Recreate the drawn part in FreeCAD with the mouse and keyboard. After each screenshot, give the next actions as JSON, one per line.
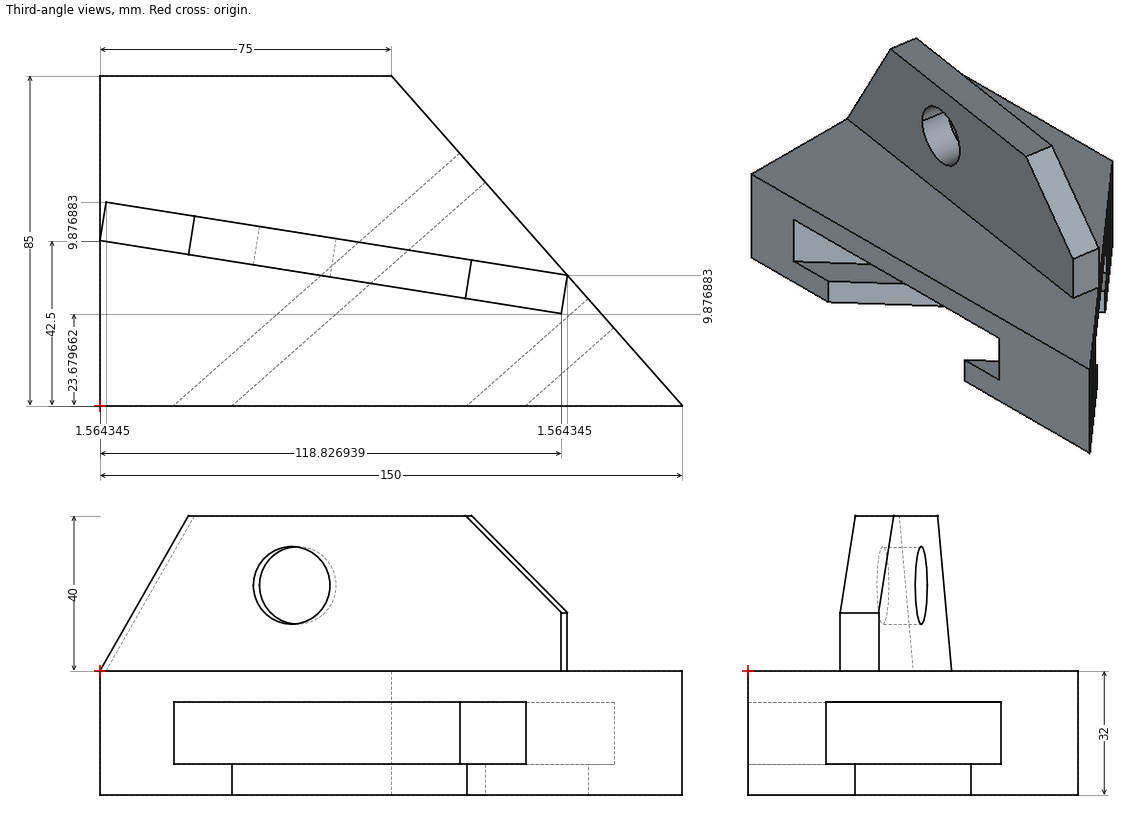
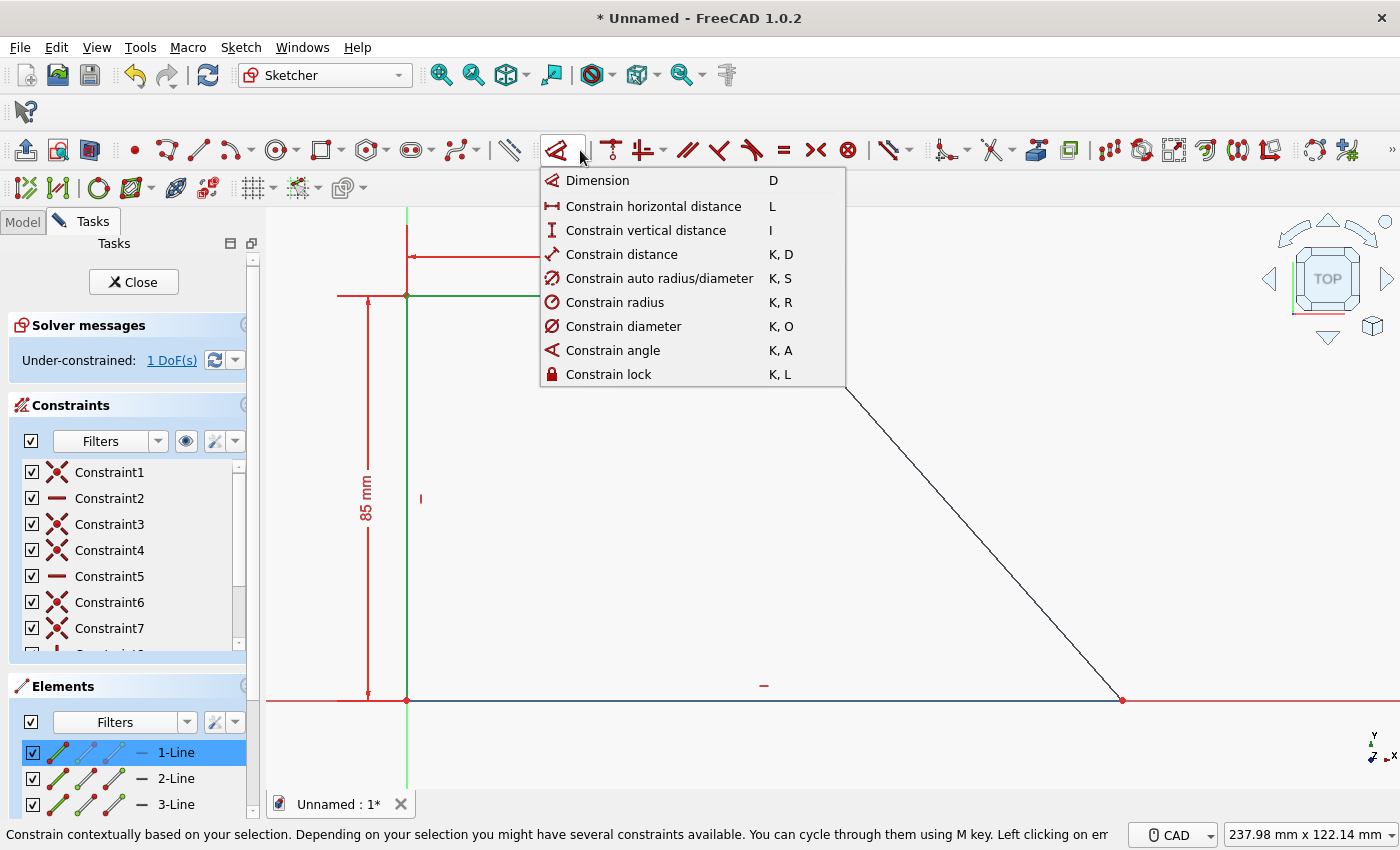
{"action": "left_click", "coordinate": [693, 206]}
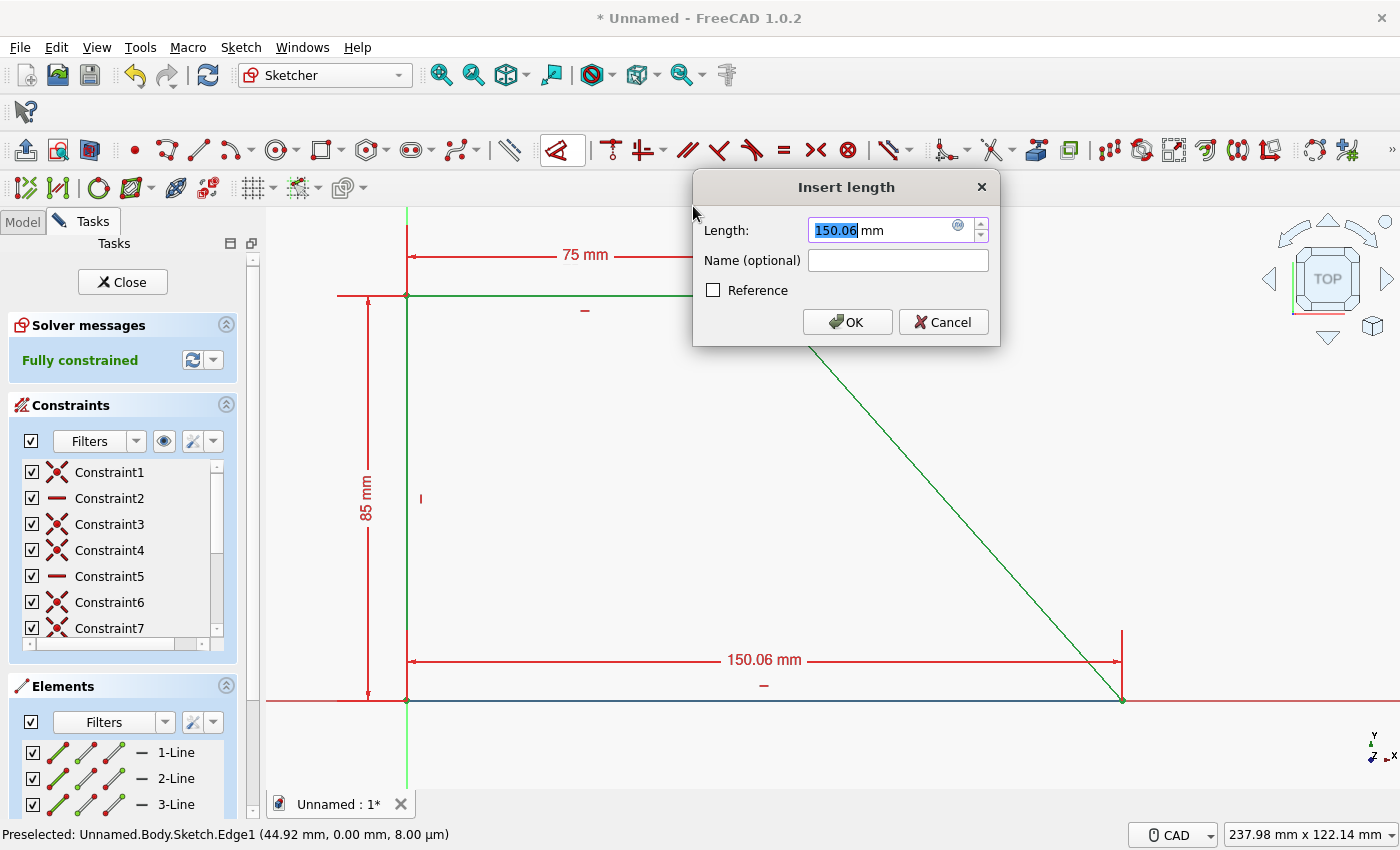
{"action": "type", "text": "150"}
{"action": "key", "text": "Return"}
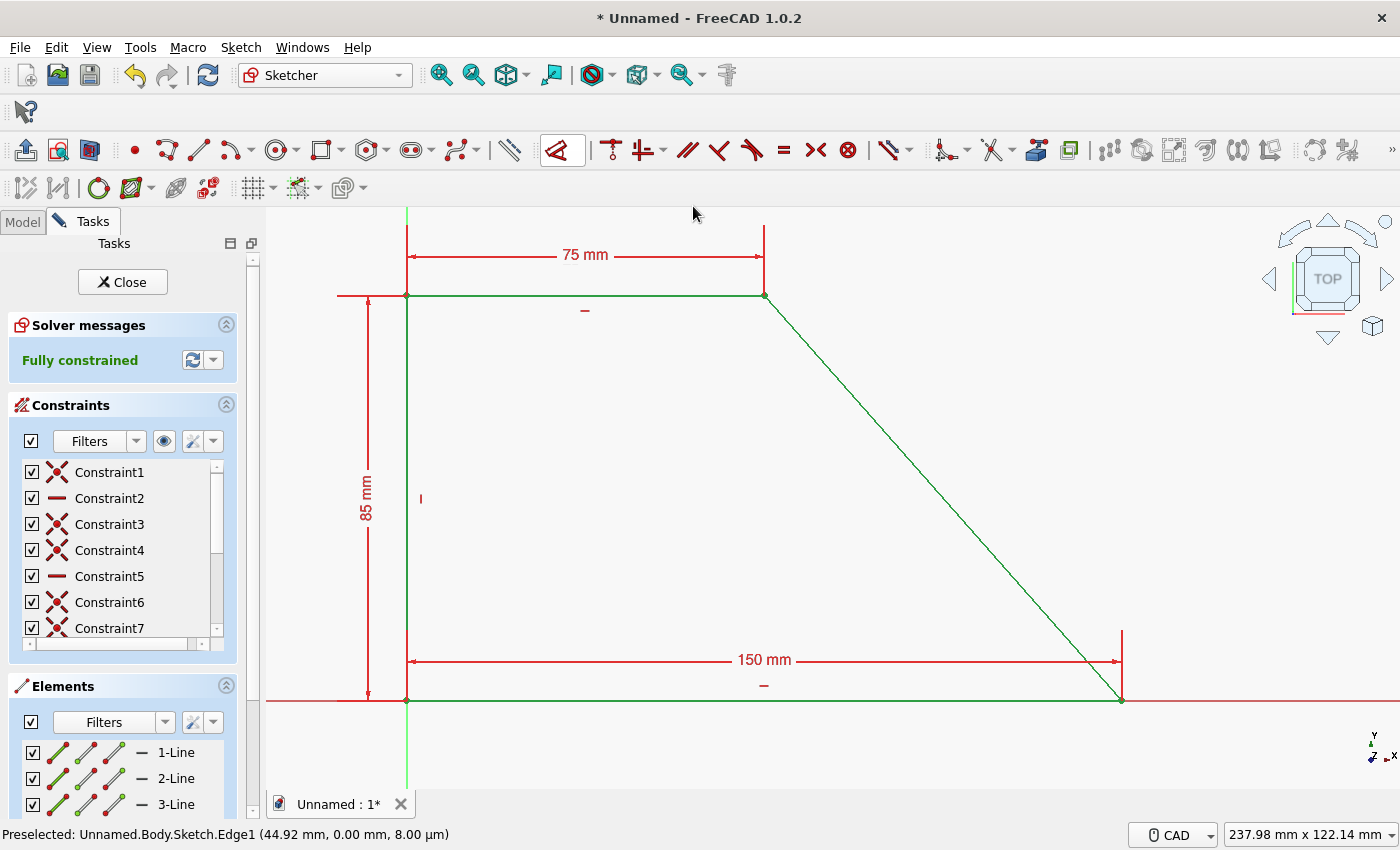
{"action": "left_click", "coordinate": [123, 282]}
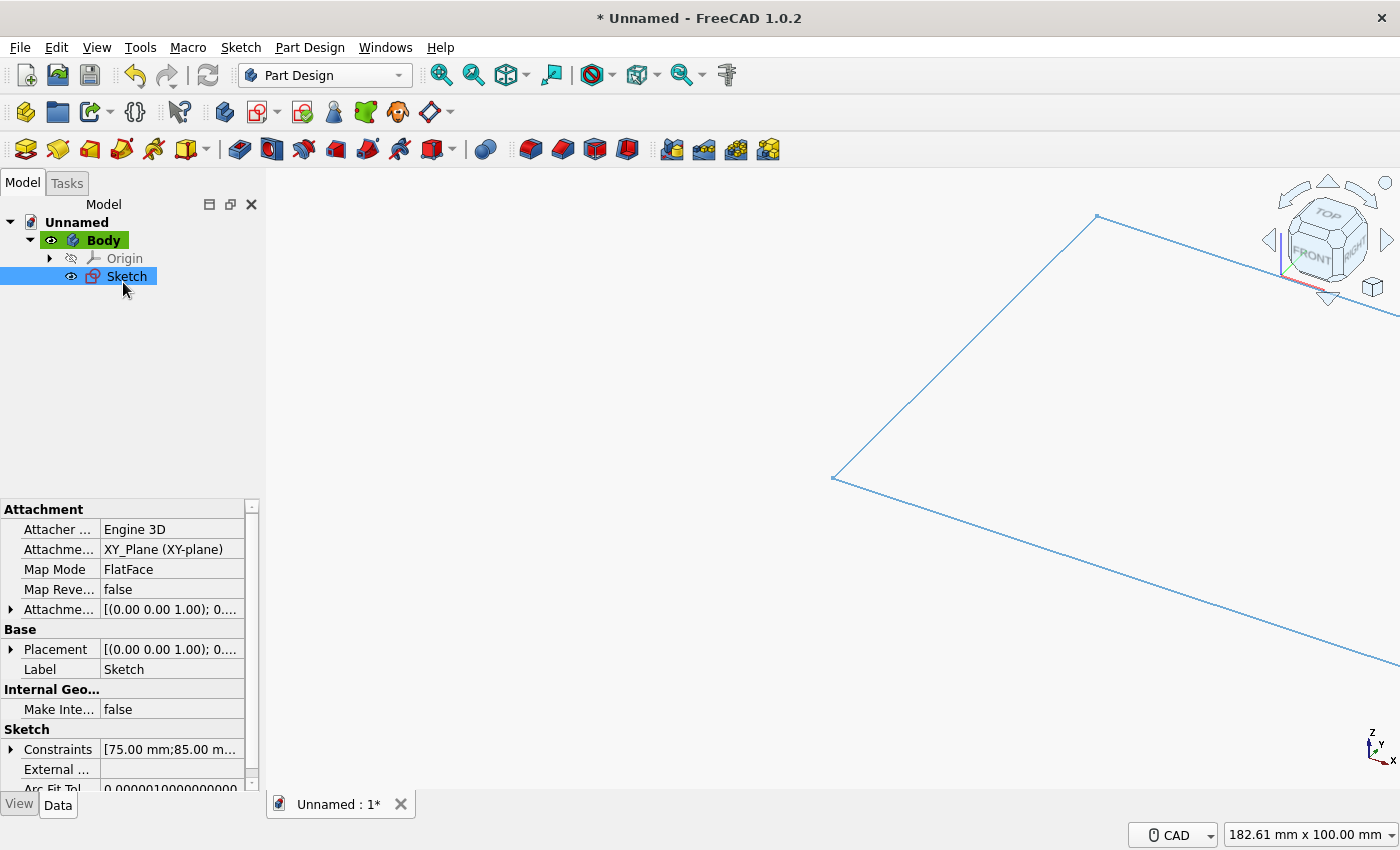
{"action": "left_click", "coordinate": [26, 150]}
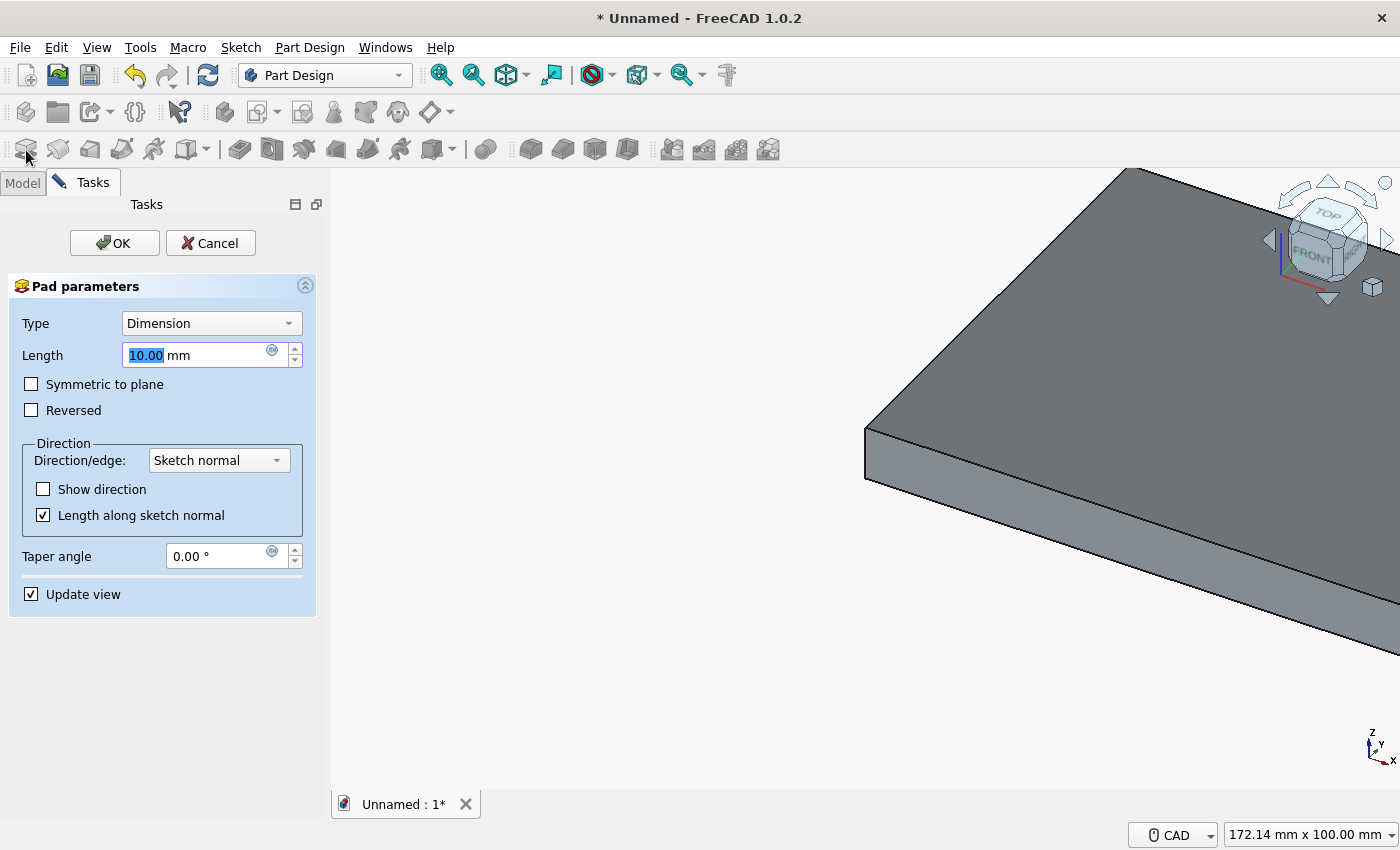
{"action": "type", "text": "32"}
{"action": "key", "text": "Tab"}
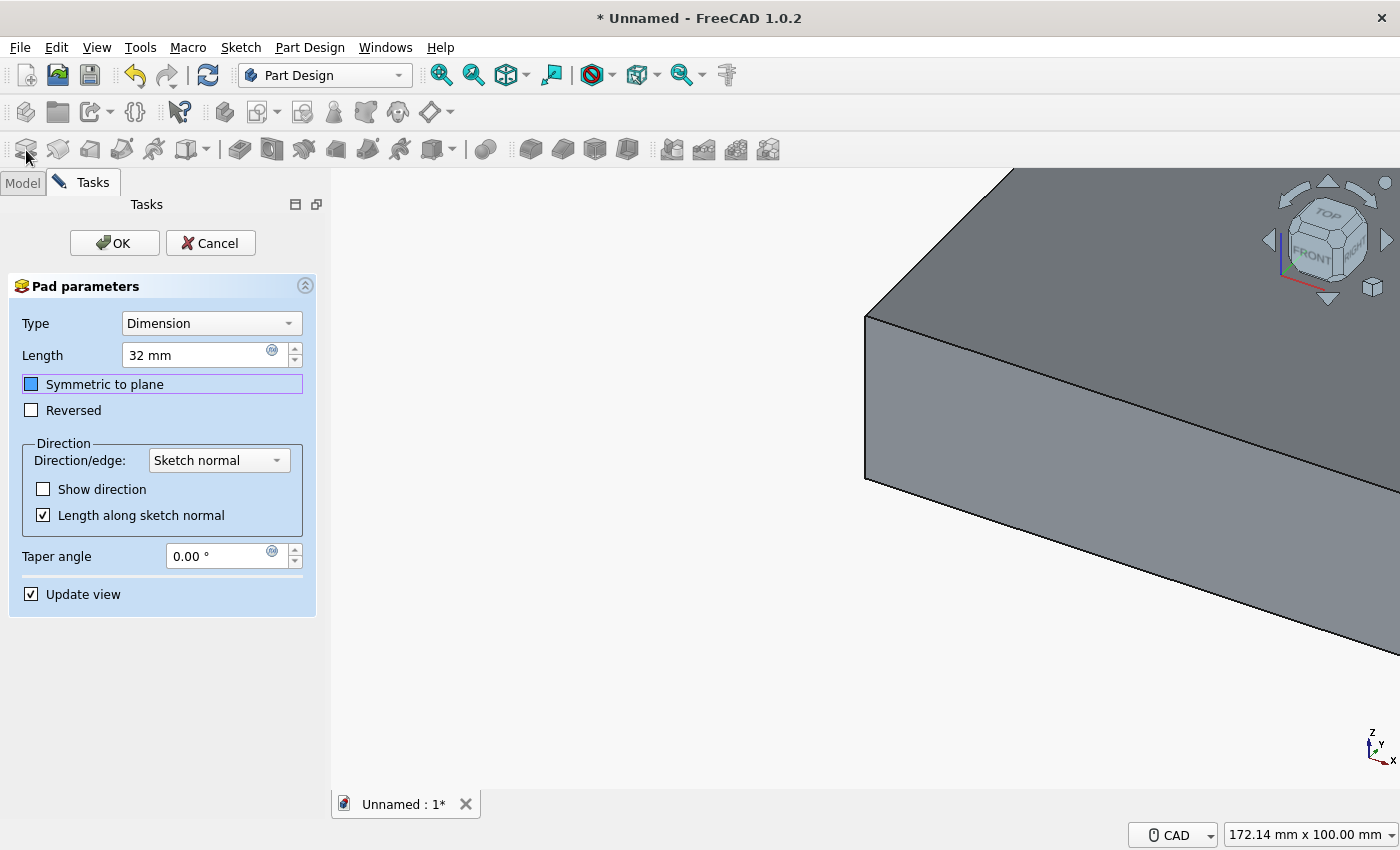
{"action": "left_click", "coordinate": [30, 410]}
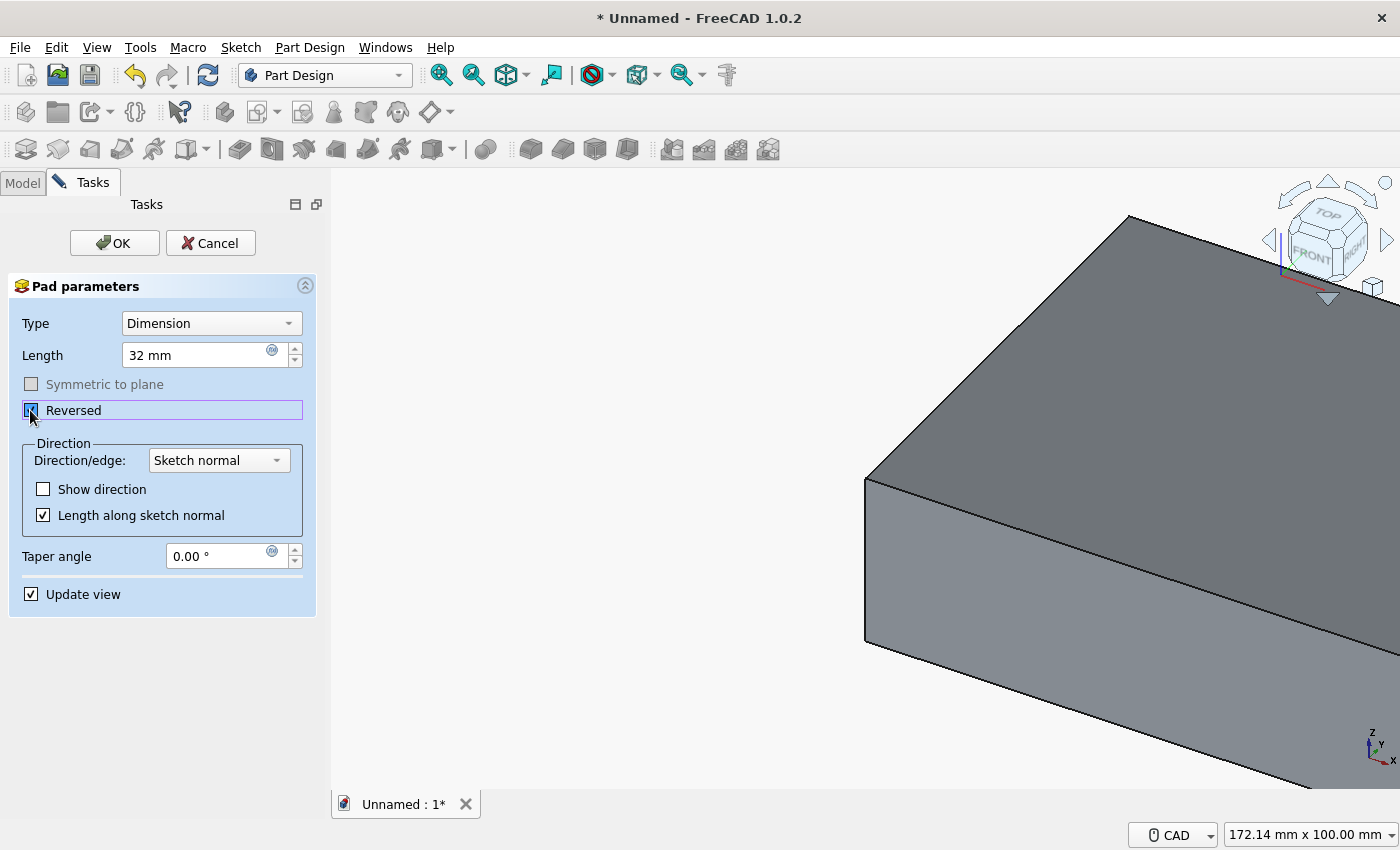
{"action": "left_click", "coordinate": [115, 243]}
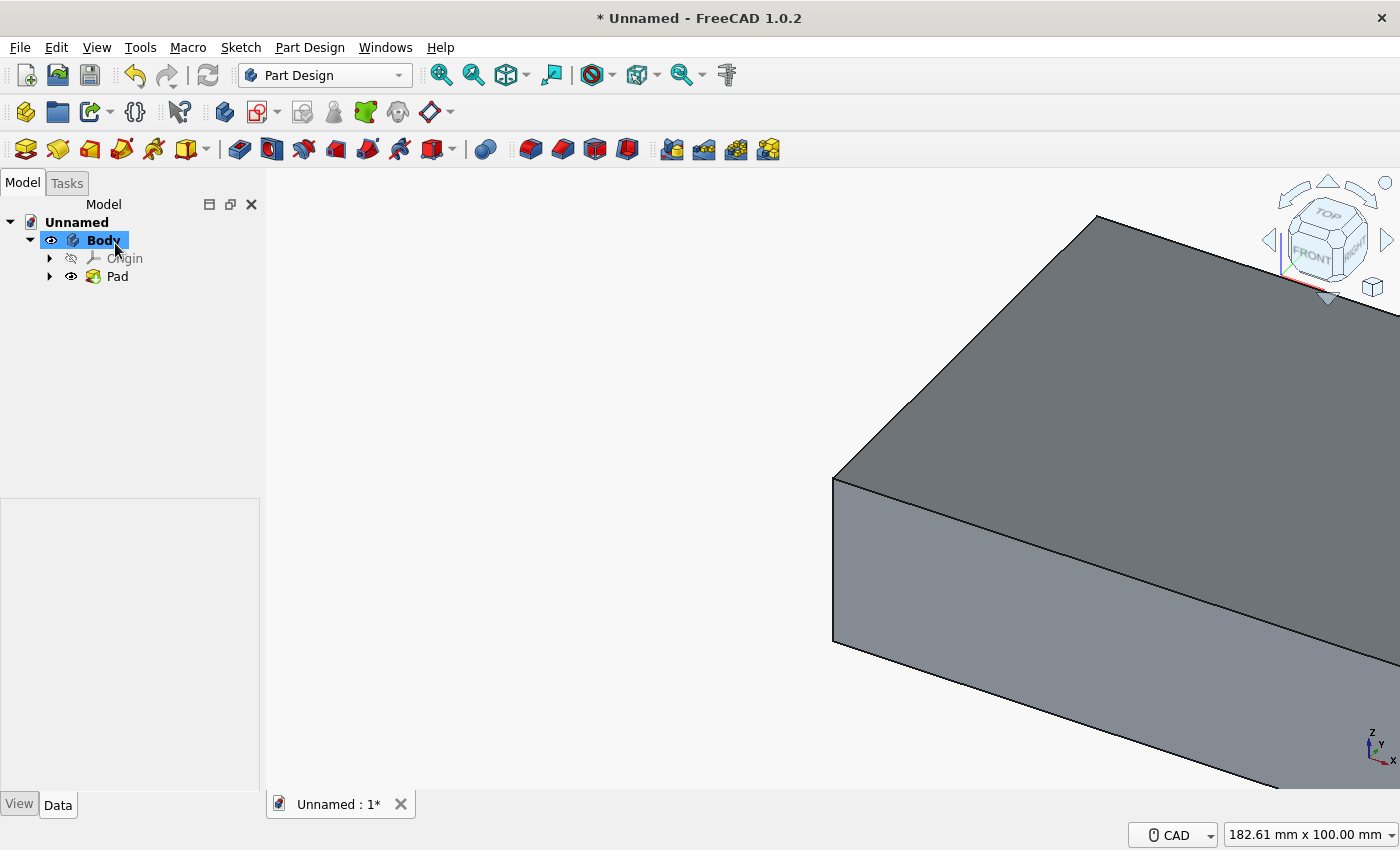
{"action": "key", "text": "v f"}